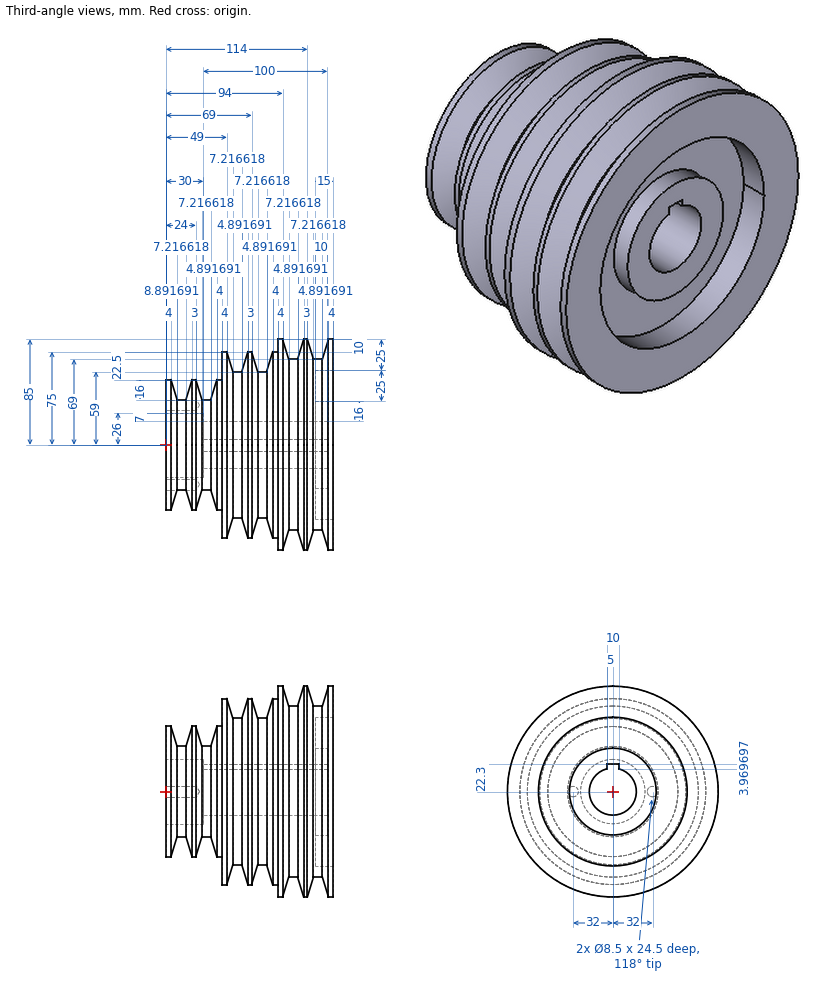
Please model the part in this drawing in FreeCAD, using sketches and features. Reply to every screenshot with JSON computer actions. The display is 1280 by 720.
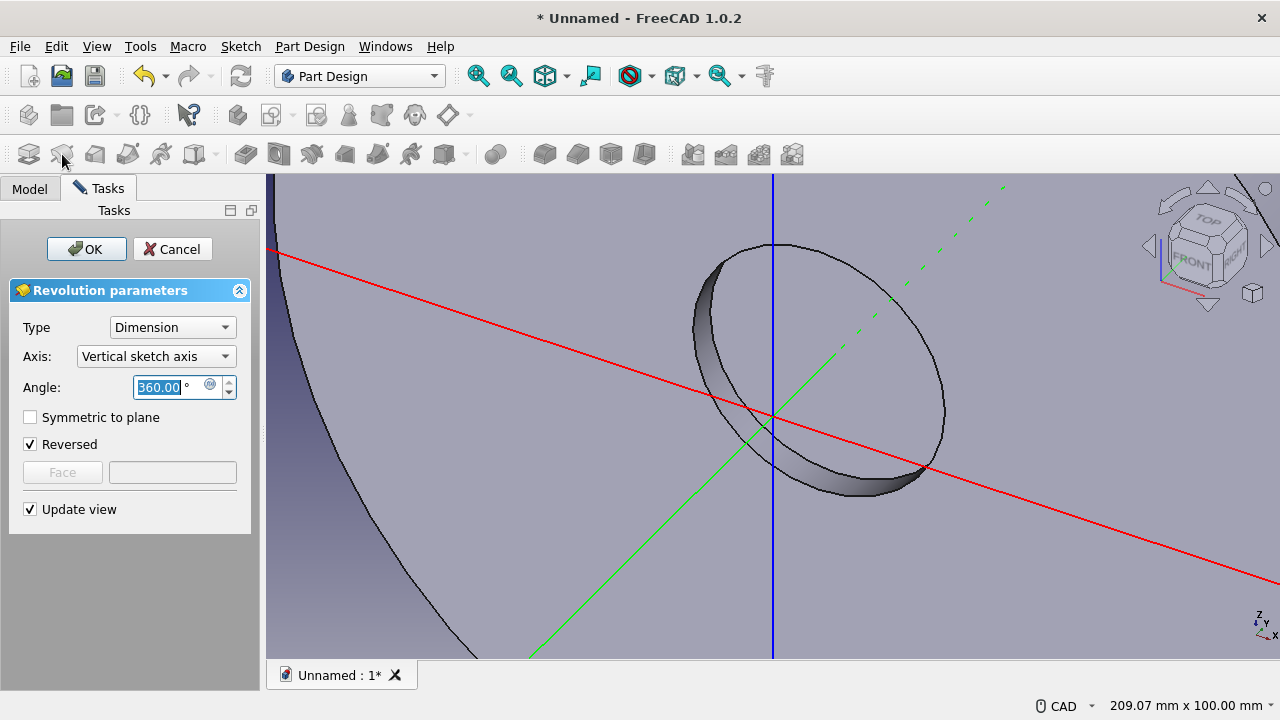
{"action": "left_click", "coordinate": [157, 356]}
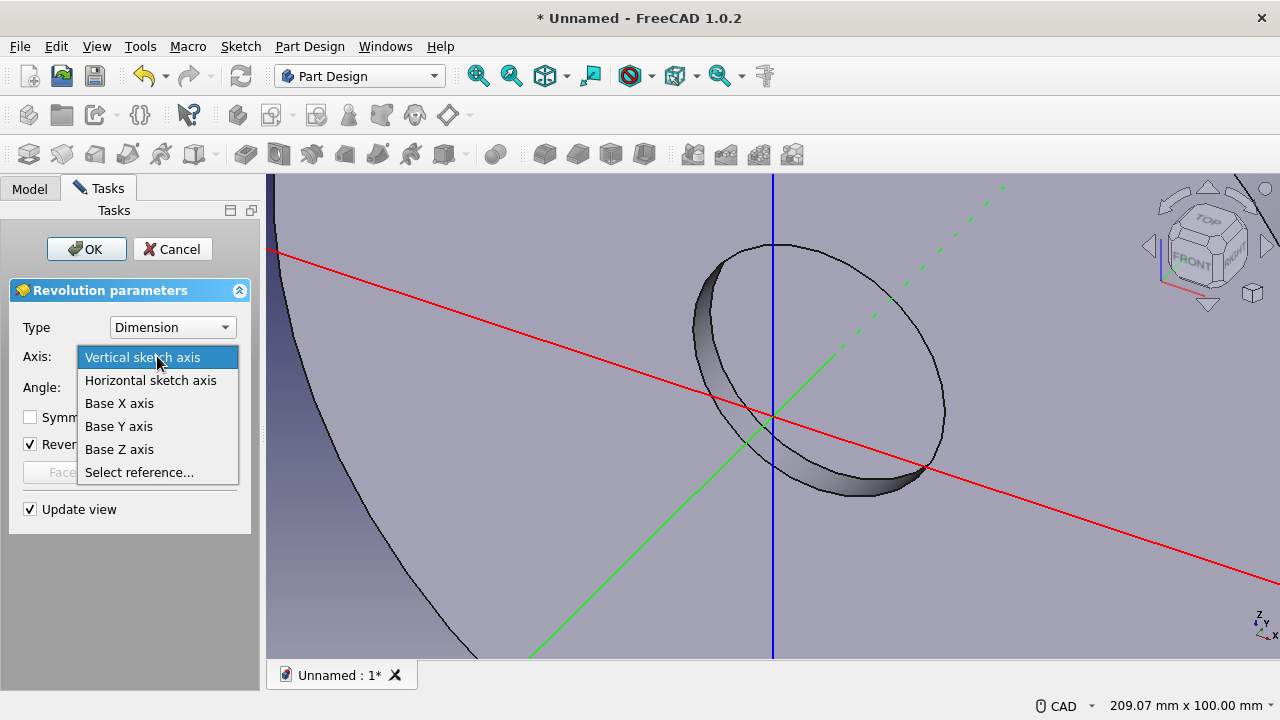
{"action": "left_click", "coordinate": [156, 380]}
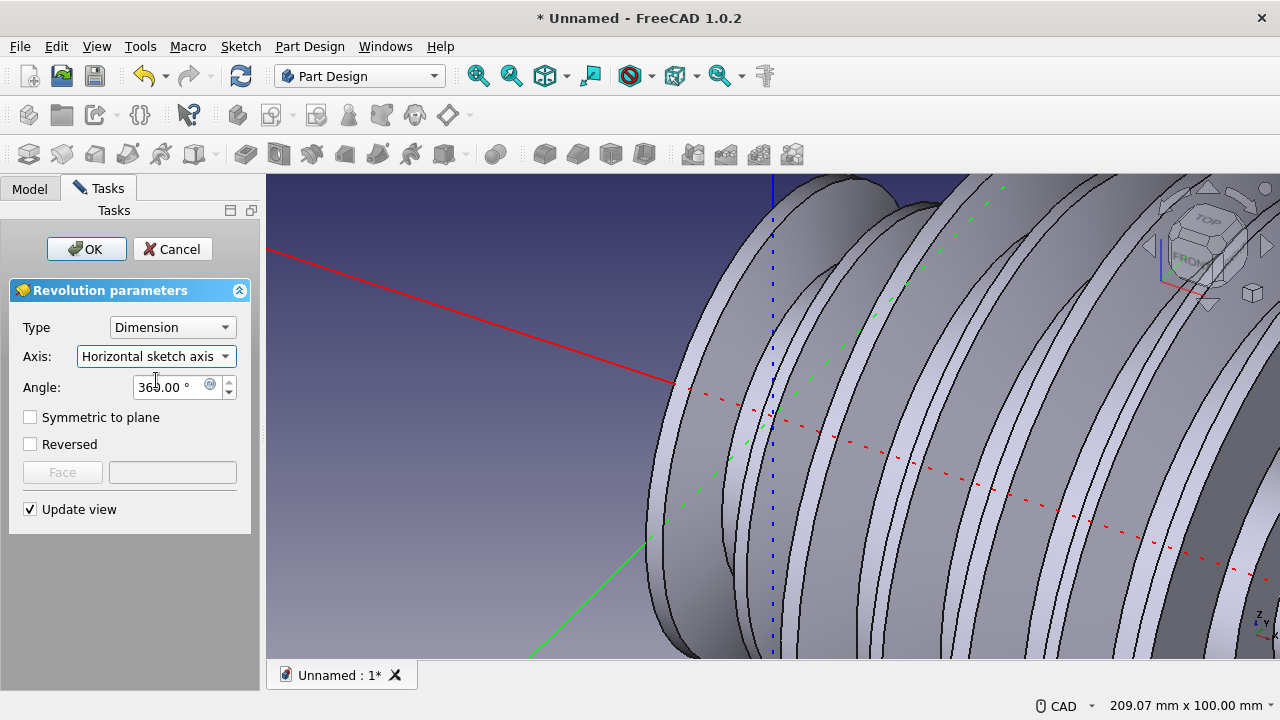
{"action": "left_click", "coordinate": [87, 249]}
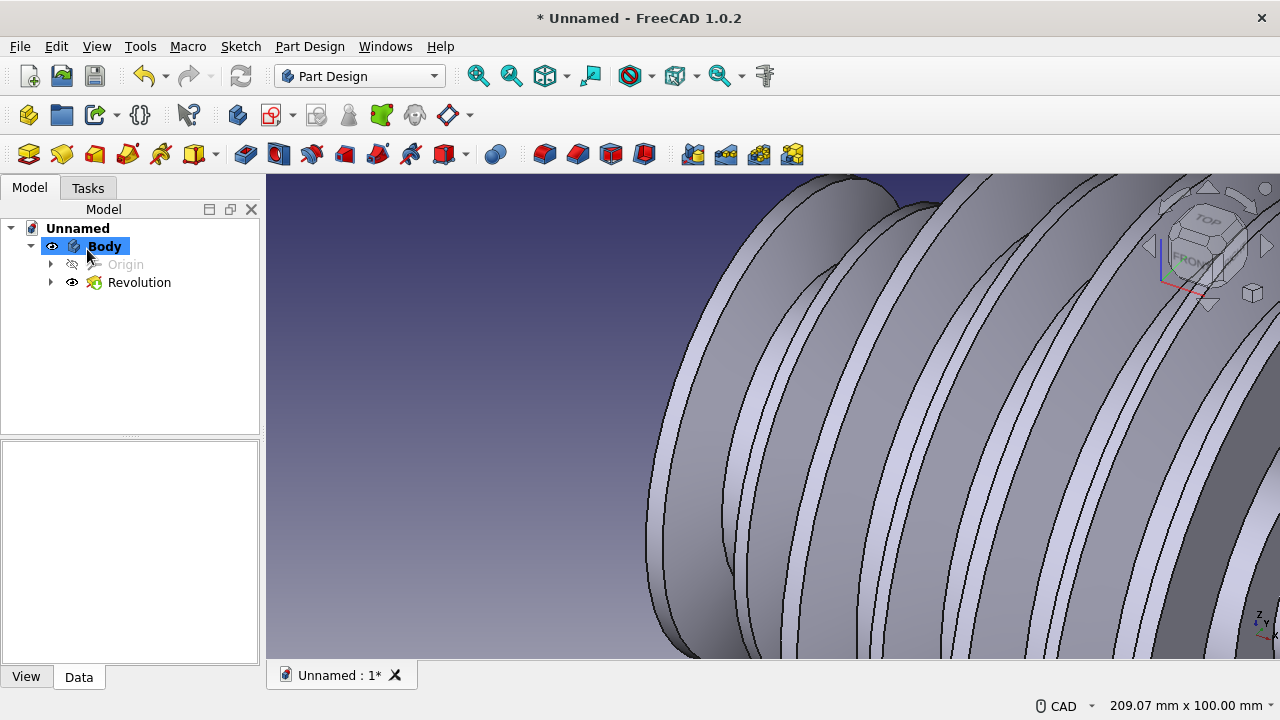
{"action": "left_click", "coordinate": [479, 76]}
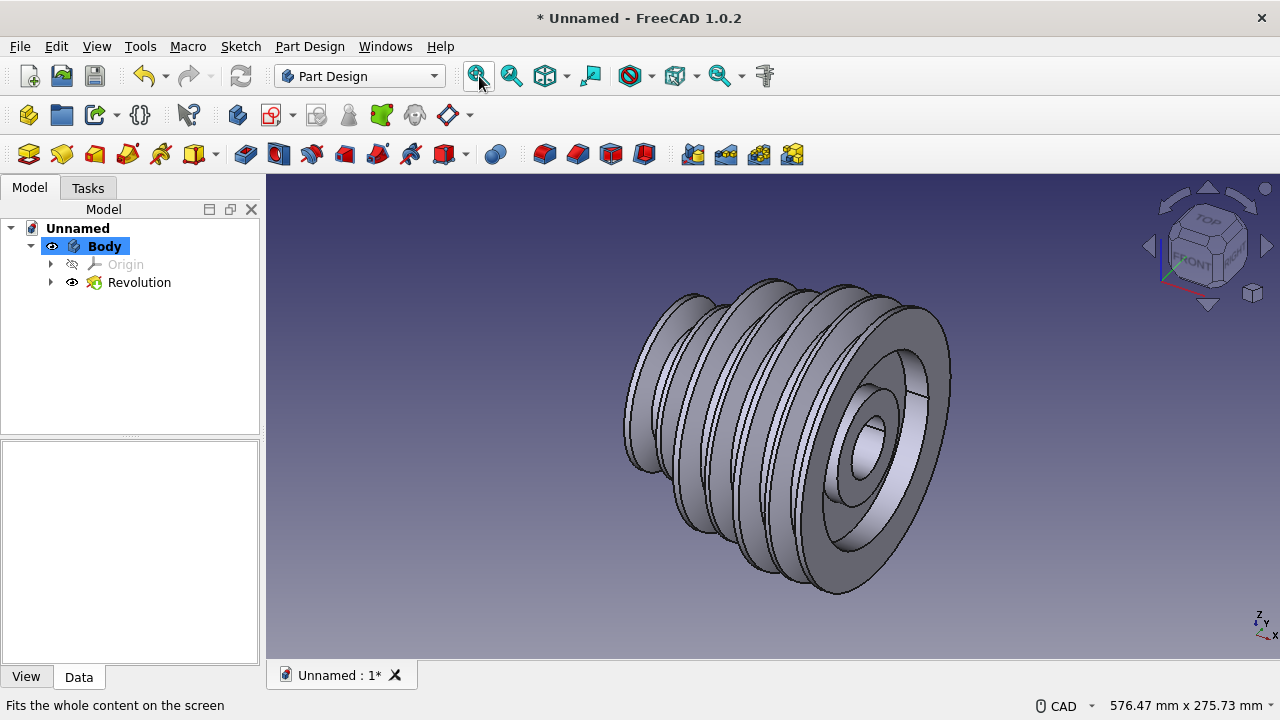
{"action": "key", "text": "6"}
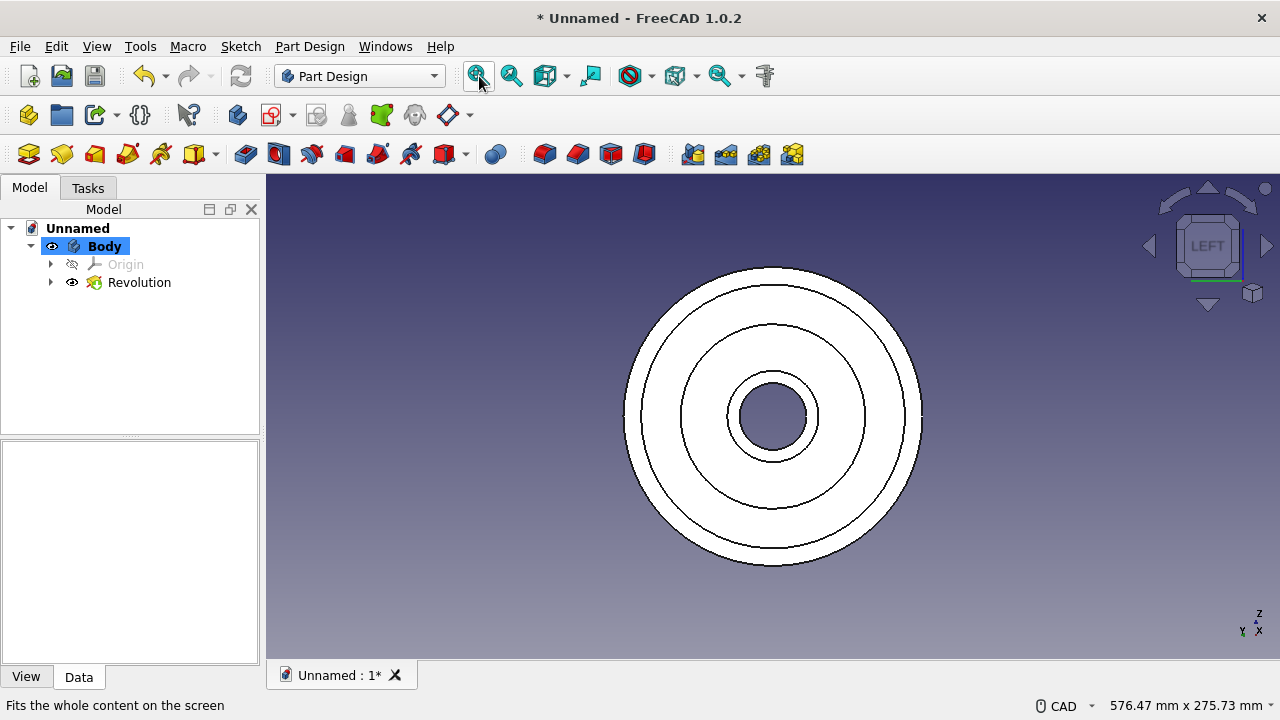
{"action": "left_click", "coordinate": [720, 468]}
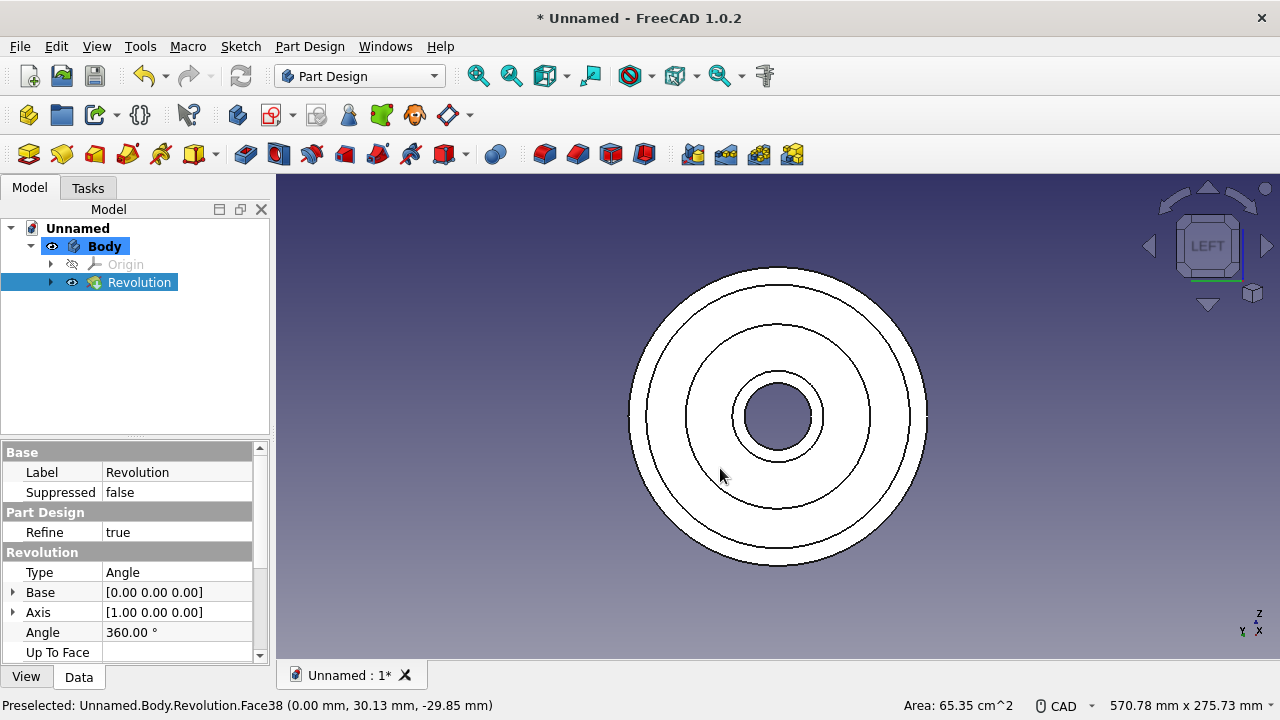
{"action": "left_click", "coordinate": [270, 116]}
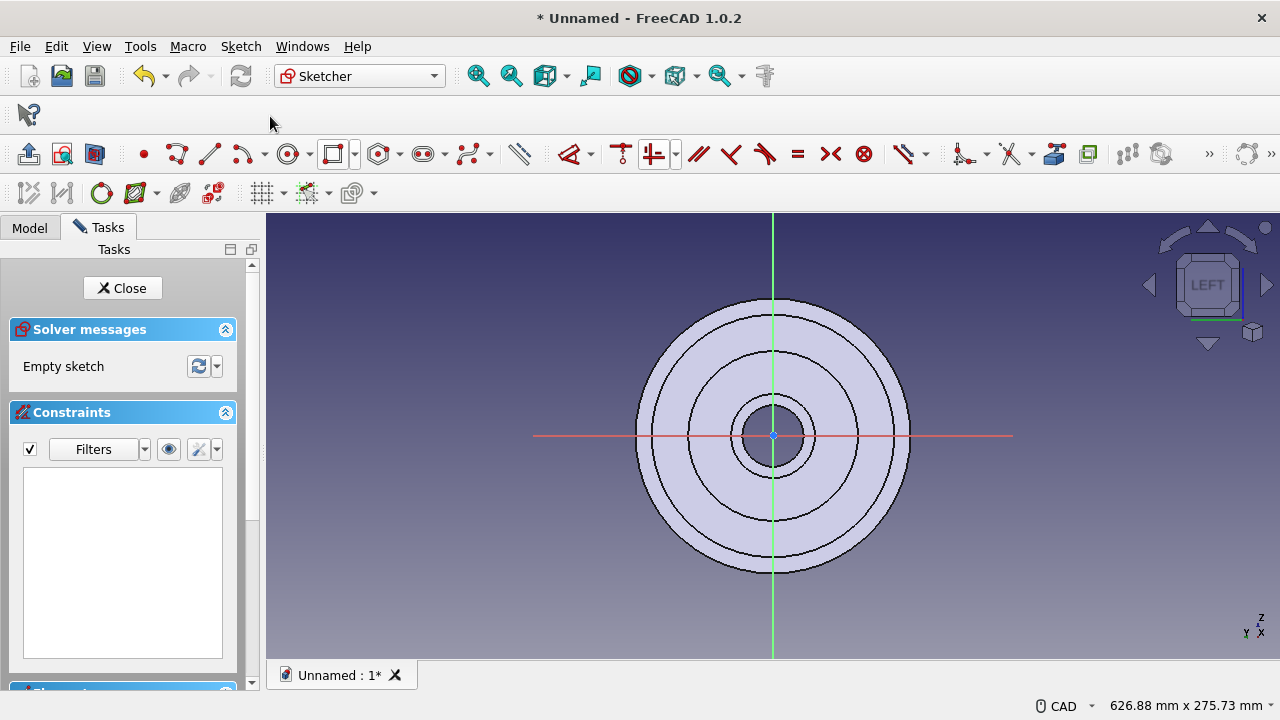
{"action": "scroll", "coordinate": [790, 436], "scroll_direction": "up", "scroll_amount": 8}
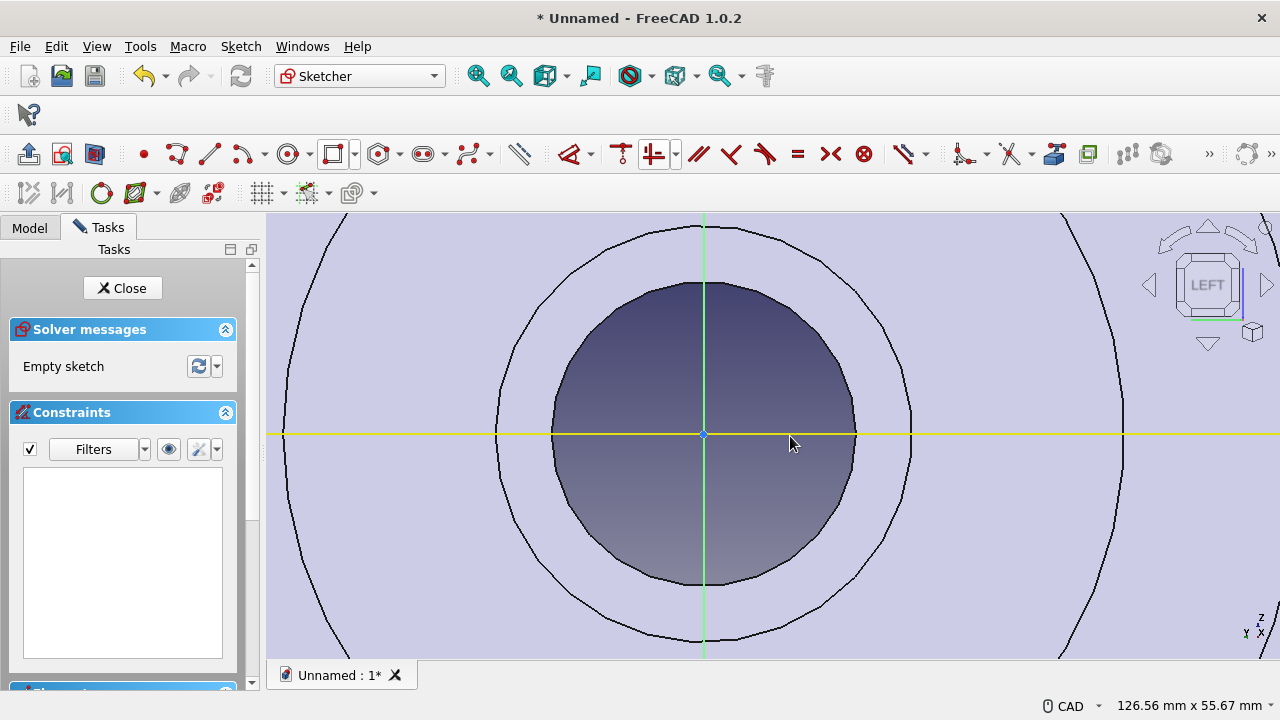
{"action": "left_click", "coordinate": [288, 154]}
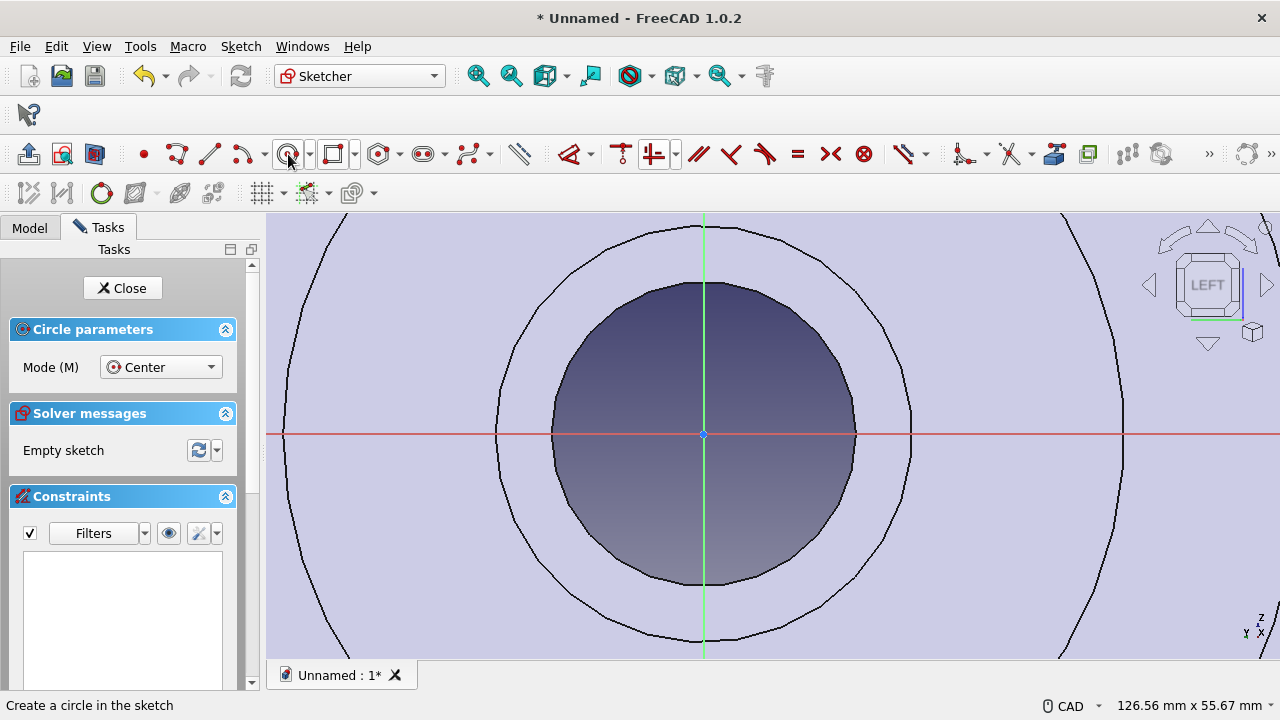
{"action": "left_click", "coordinate": [447, 434]}
{"action": "mouse_move", "coordinate": [471, 410]}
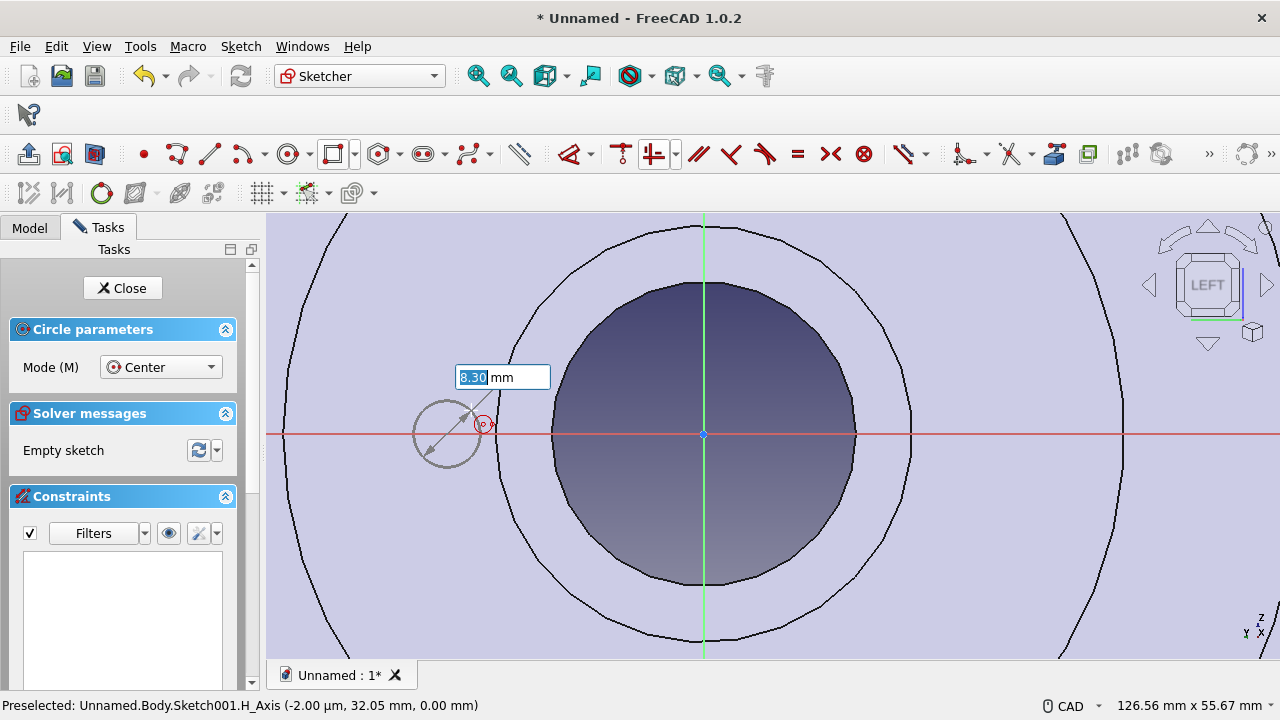
{"action": "type", "text": "8.5"}
{"action": "key", "text": "Return"}